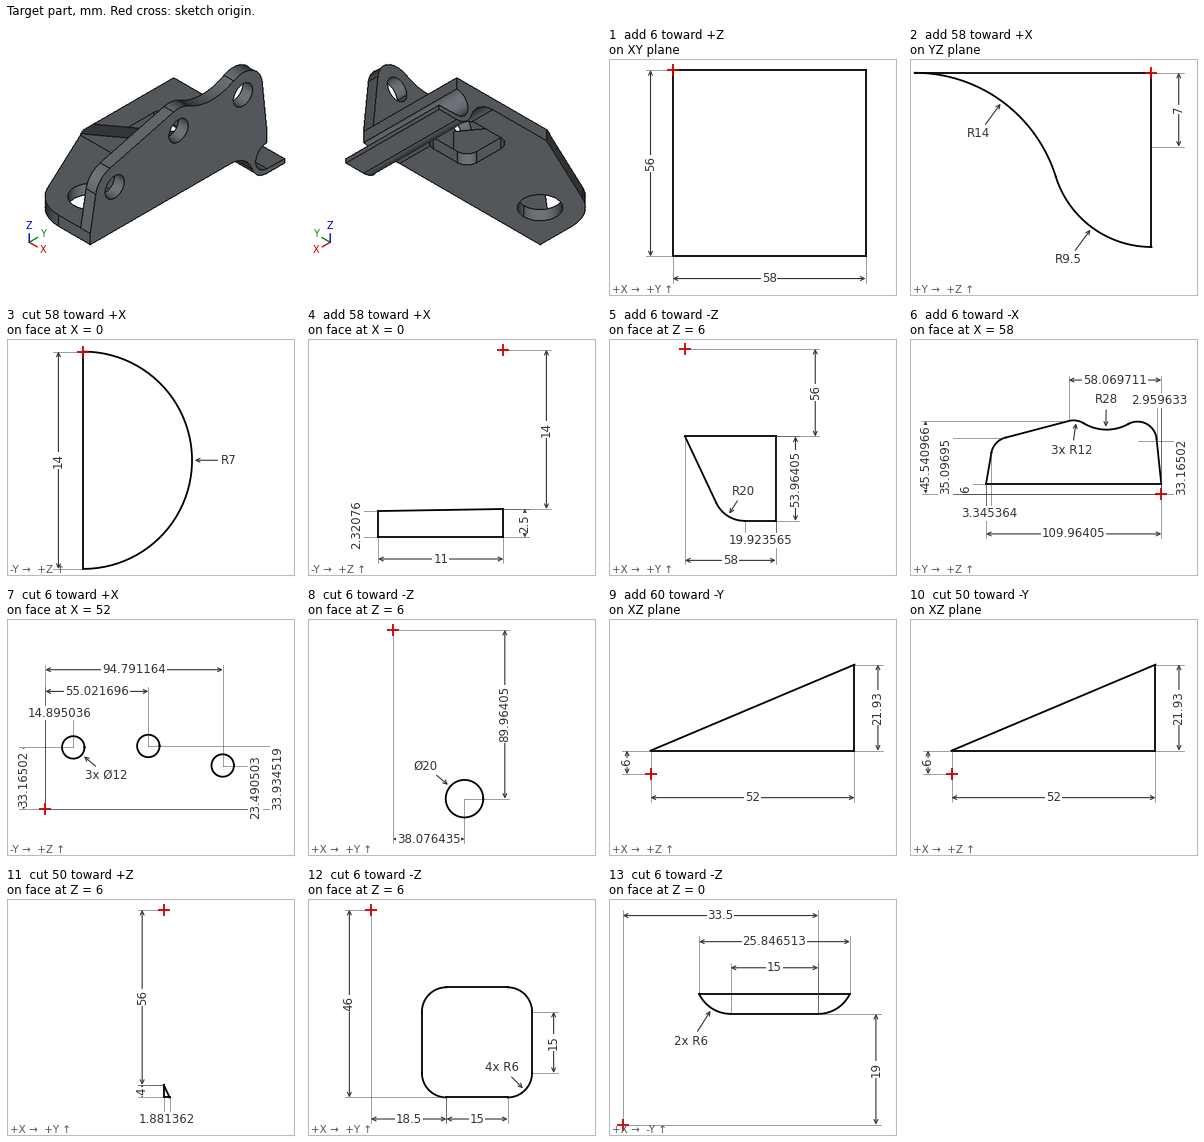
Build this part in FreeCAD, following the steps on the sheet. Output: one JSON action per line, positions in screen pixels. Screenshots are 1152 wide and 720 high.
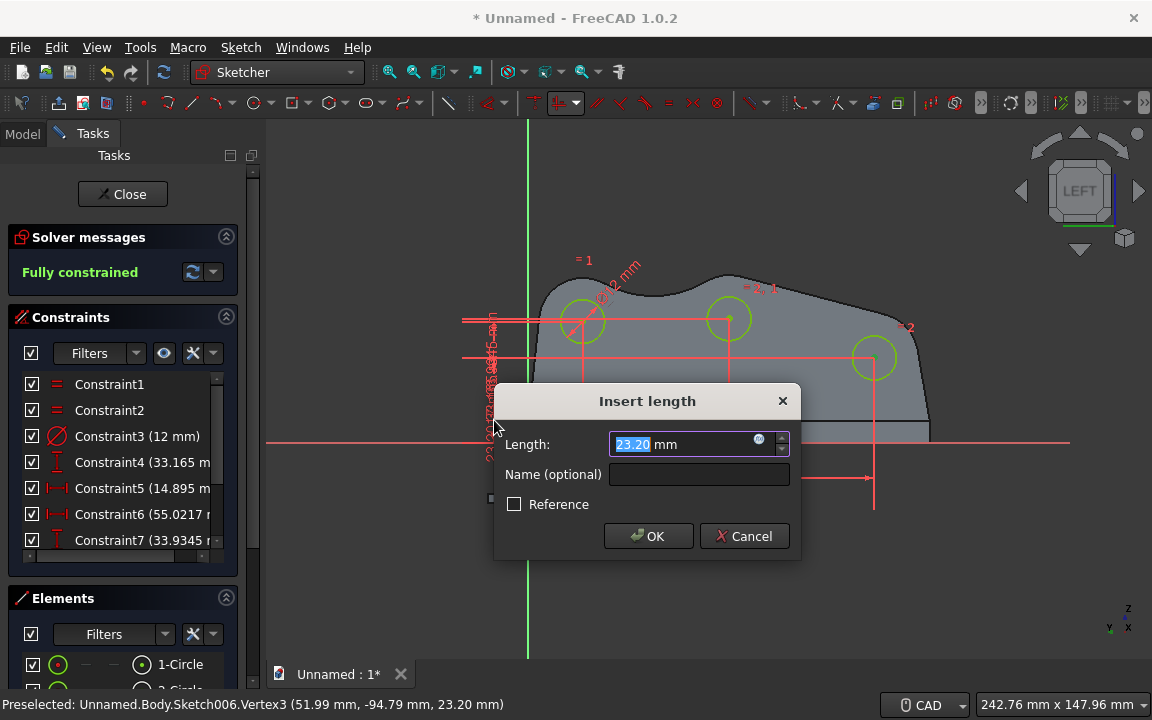
{"action": "type", "text": "23.490503"}
{"action": "key", "text": "Return"}
{"action": "key", "text": "Escape"}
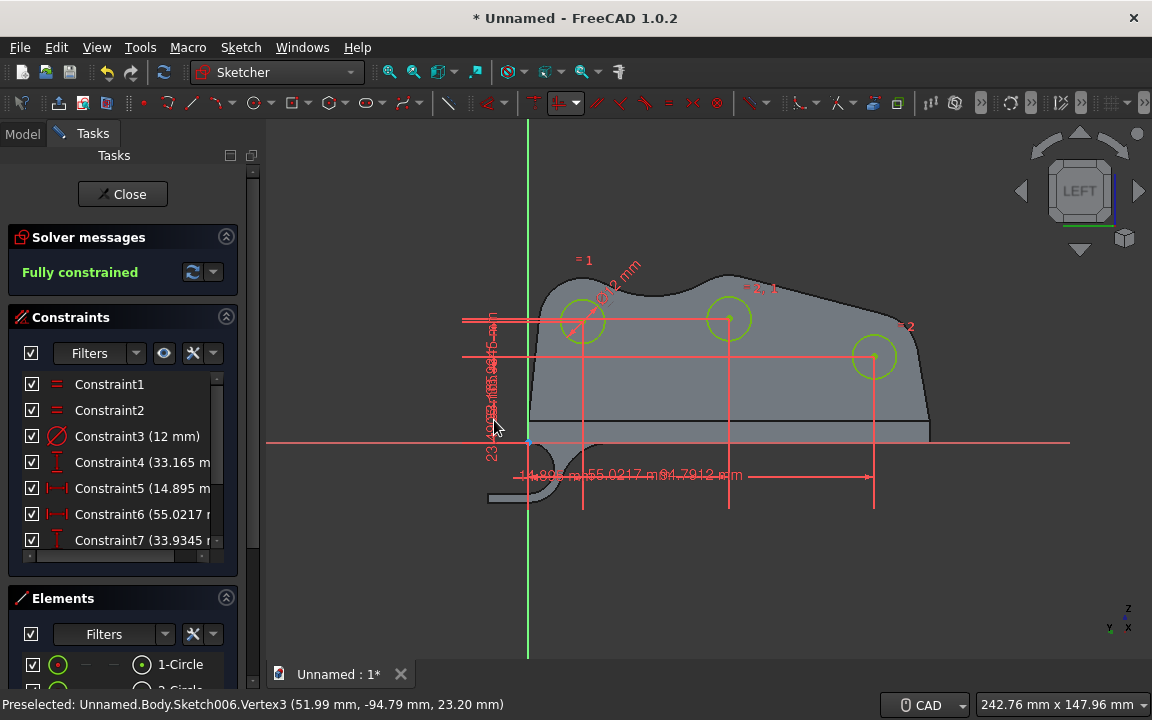
{"action": "left_click", "coordinate": [123, 194]}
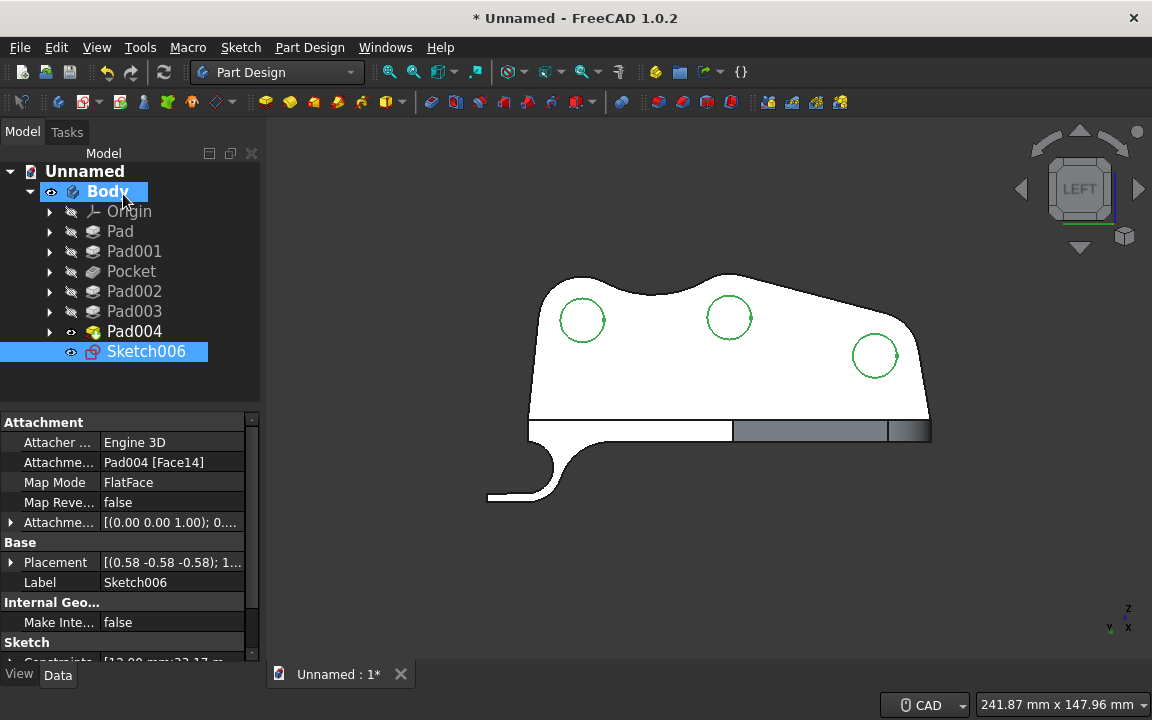
{"action": "left_click", "coordinate": [432, 102]}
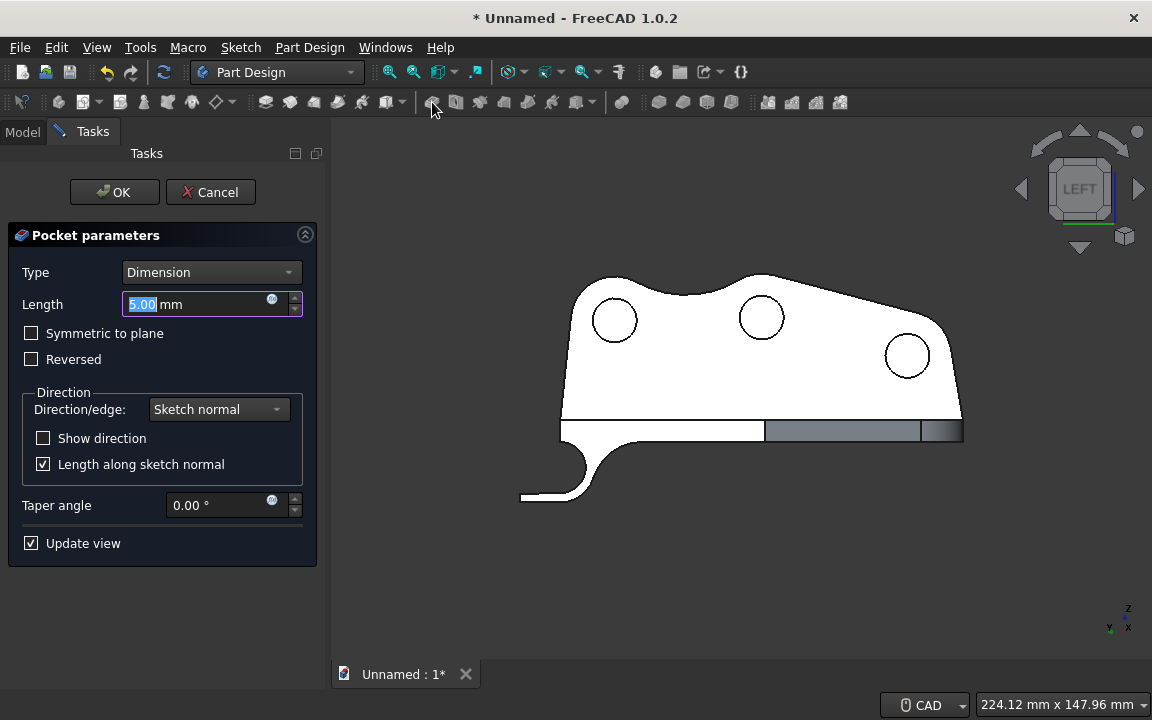
{"action": "type", "text": "6"}
{"action": "key", "text": "Tab"}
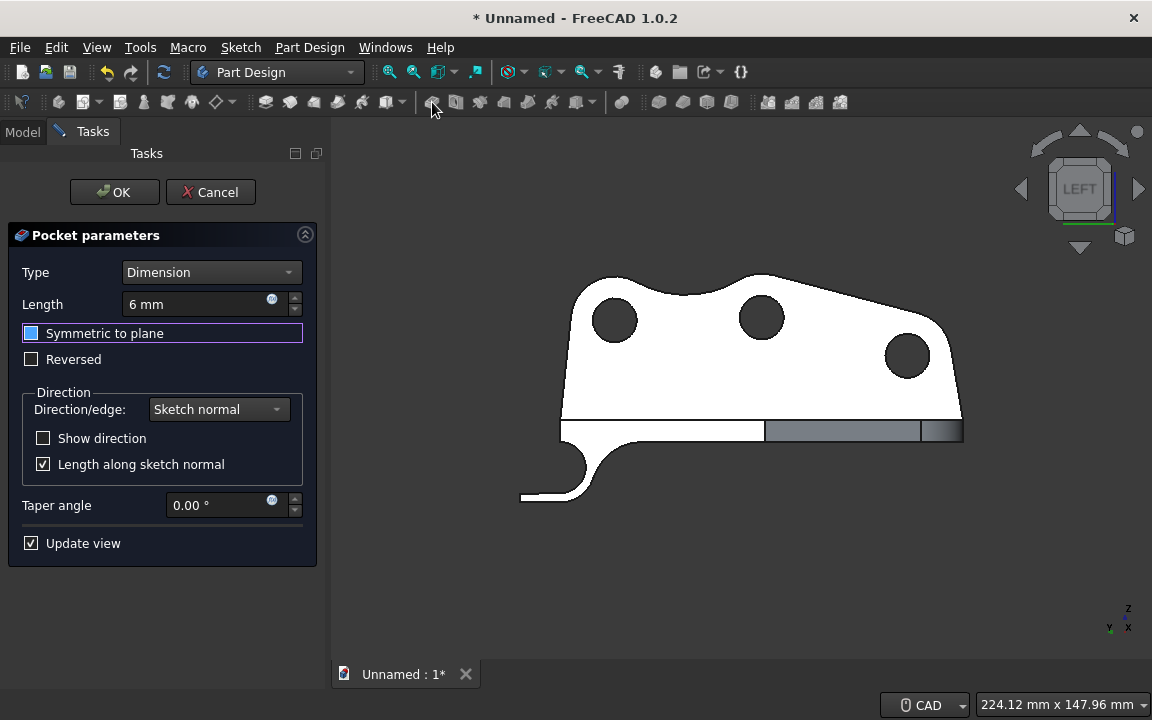
{"action": "left_click", "coordinate": [115, 192]}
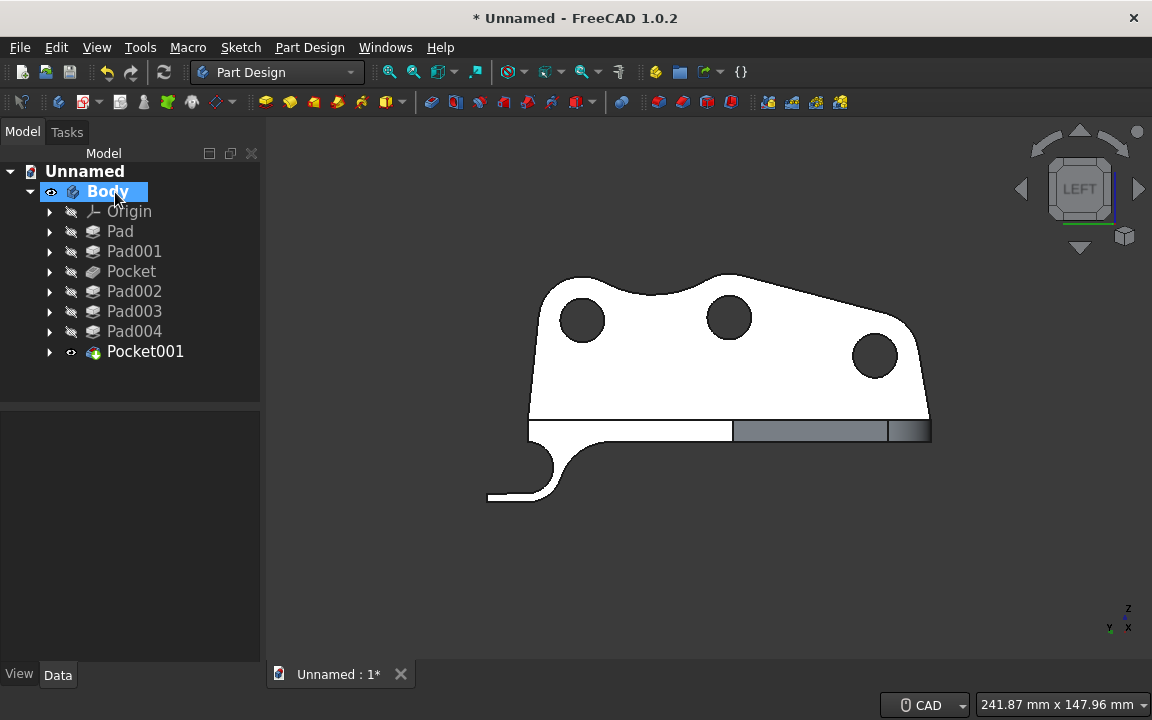
{"action": "key", "text": "0"}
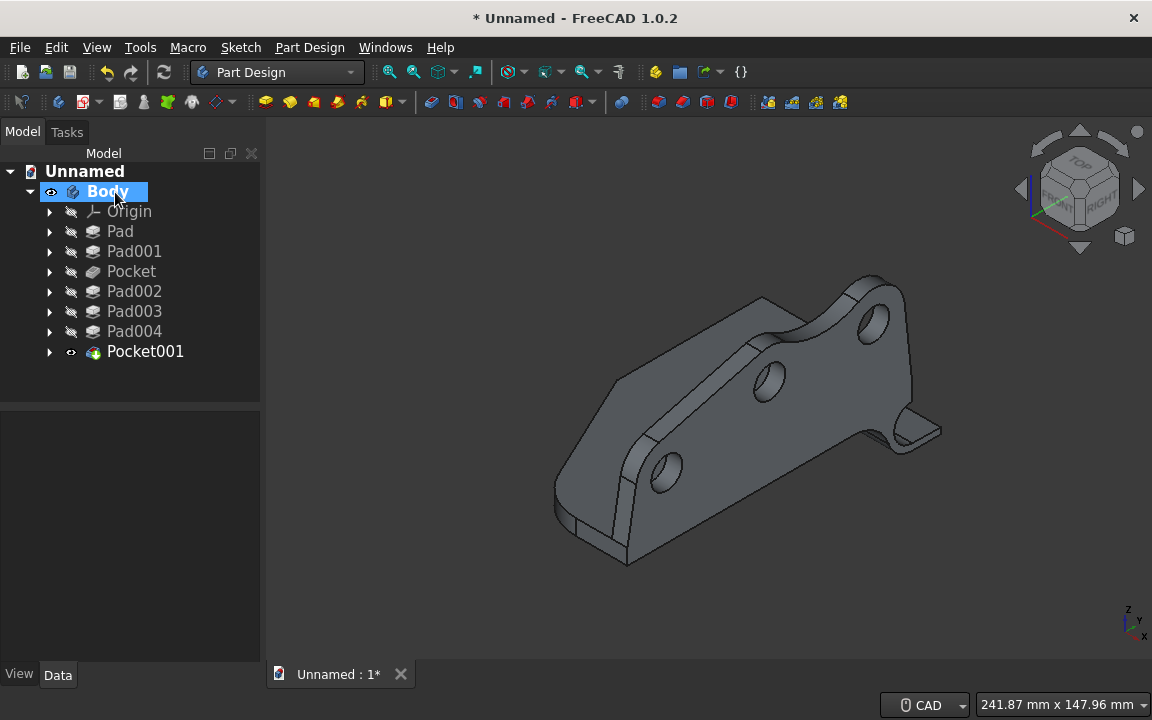
{"action": "key", "text": "2"}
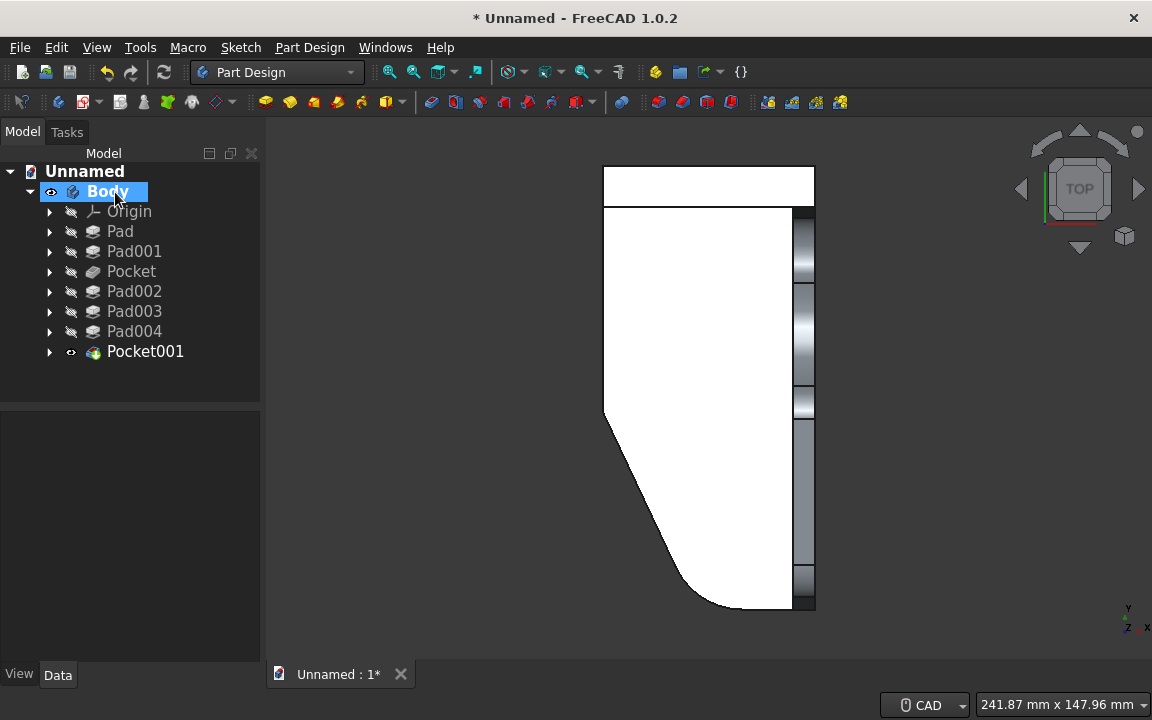
{"action": "left_click", "coordinate": [698, 350]}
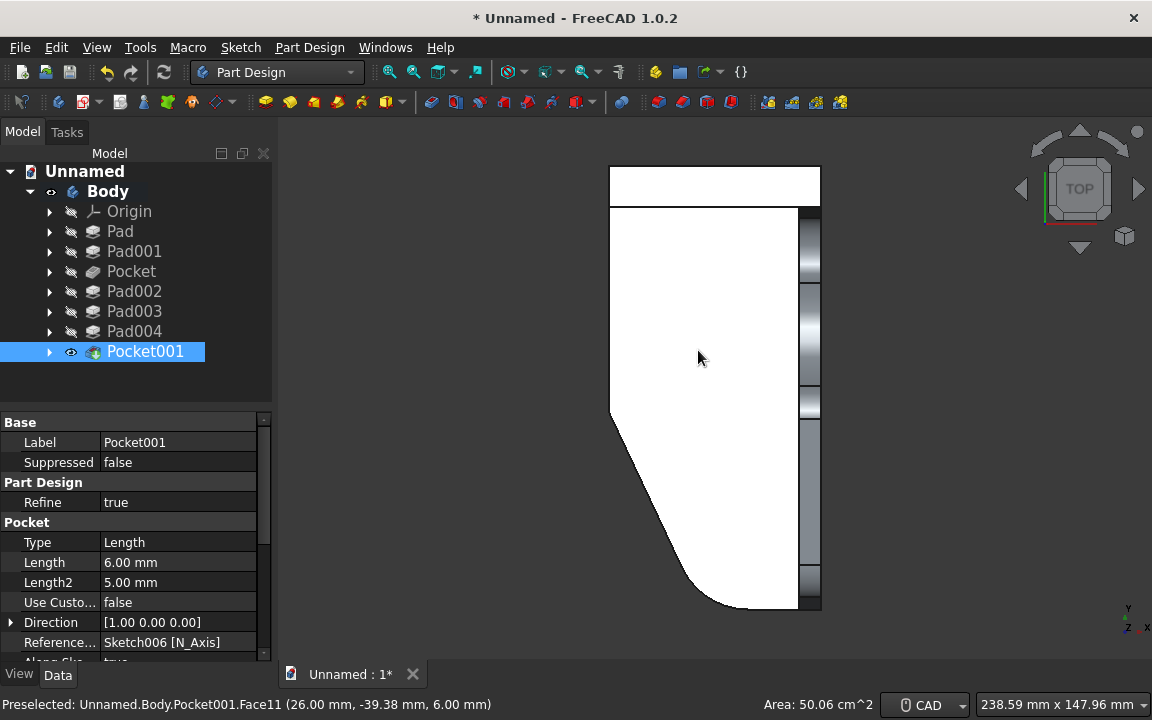
{"action": "left_click", "coordinate": [84, 102]}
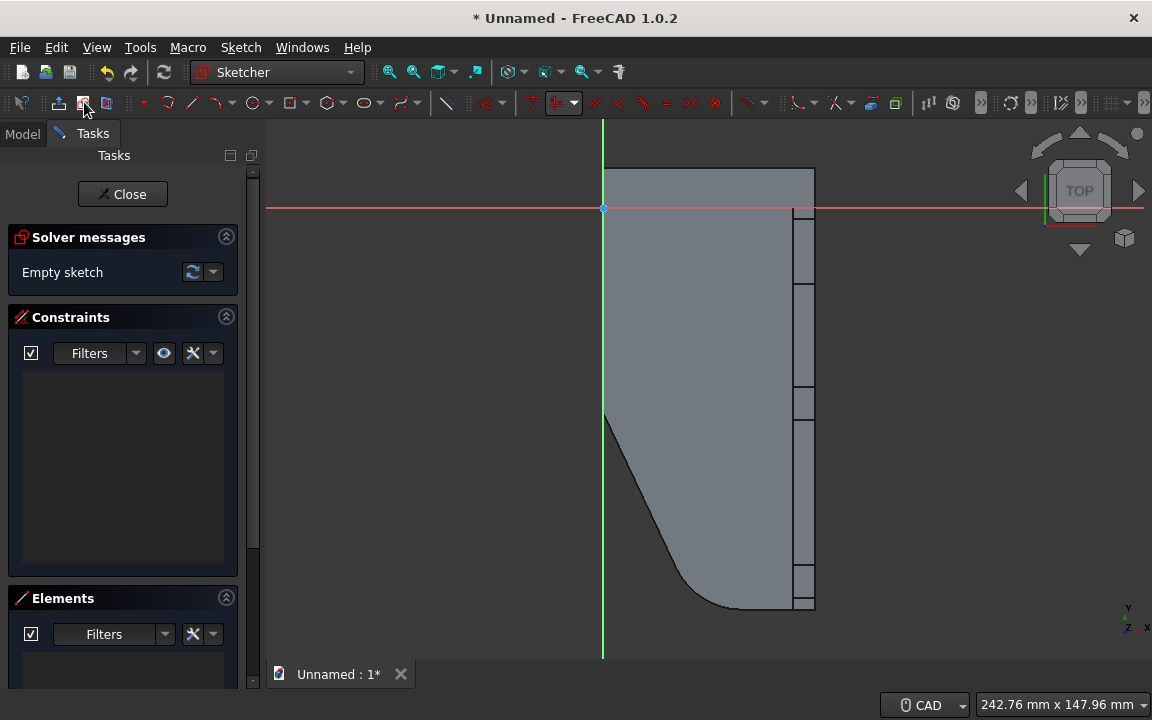
{"action": "left_click", "coordinate": [108, 104]}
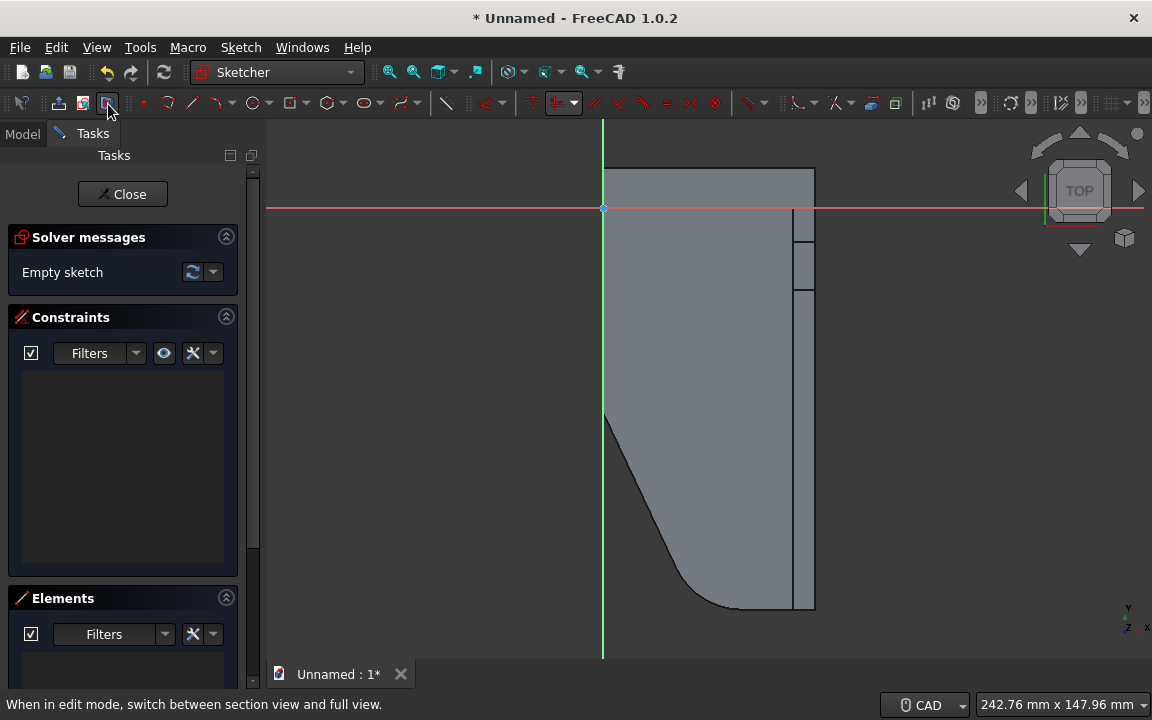
{"action": "scroll", "coordinate": [768, 574], "scroll_direction": "up", "scroll_amount": 8}